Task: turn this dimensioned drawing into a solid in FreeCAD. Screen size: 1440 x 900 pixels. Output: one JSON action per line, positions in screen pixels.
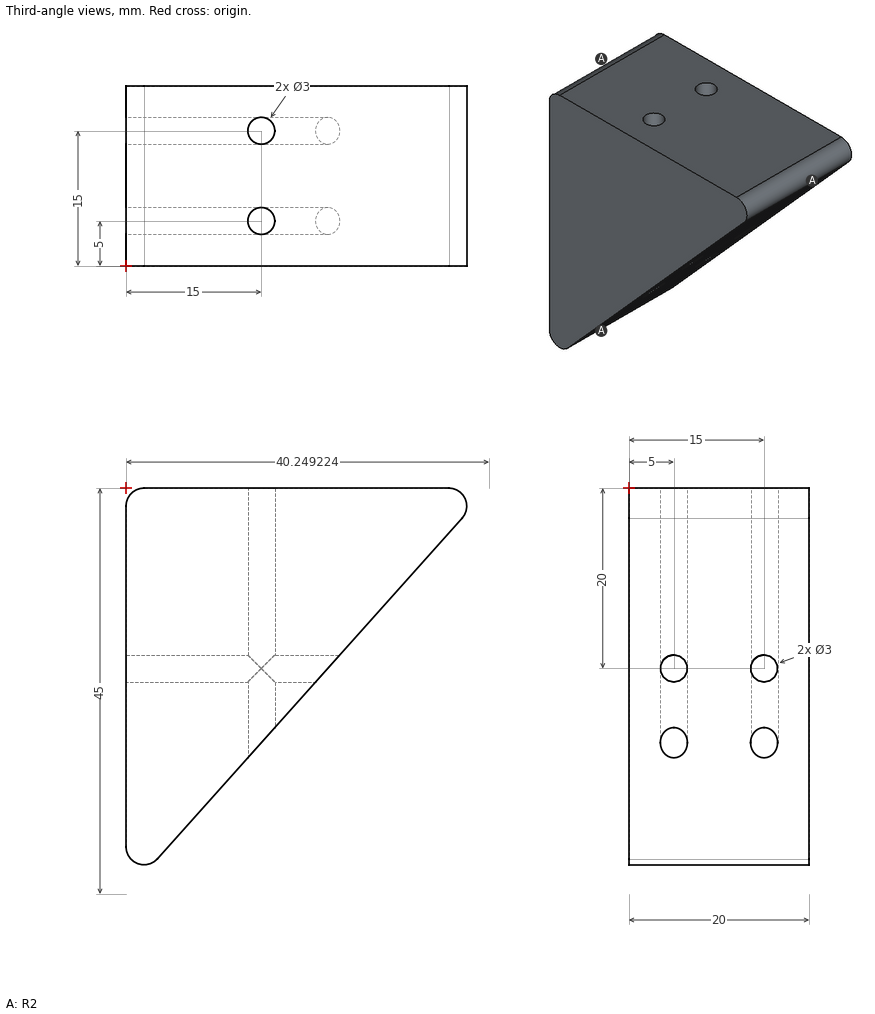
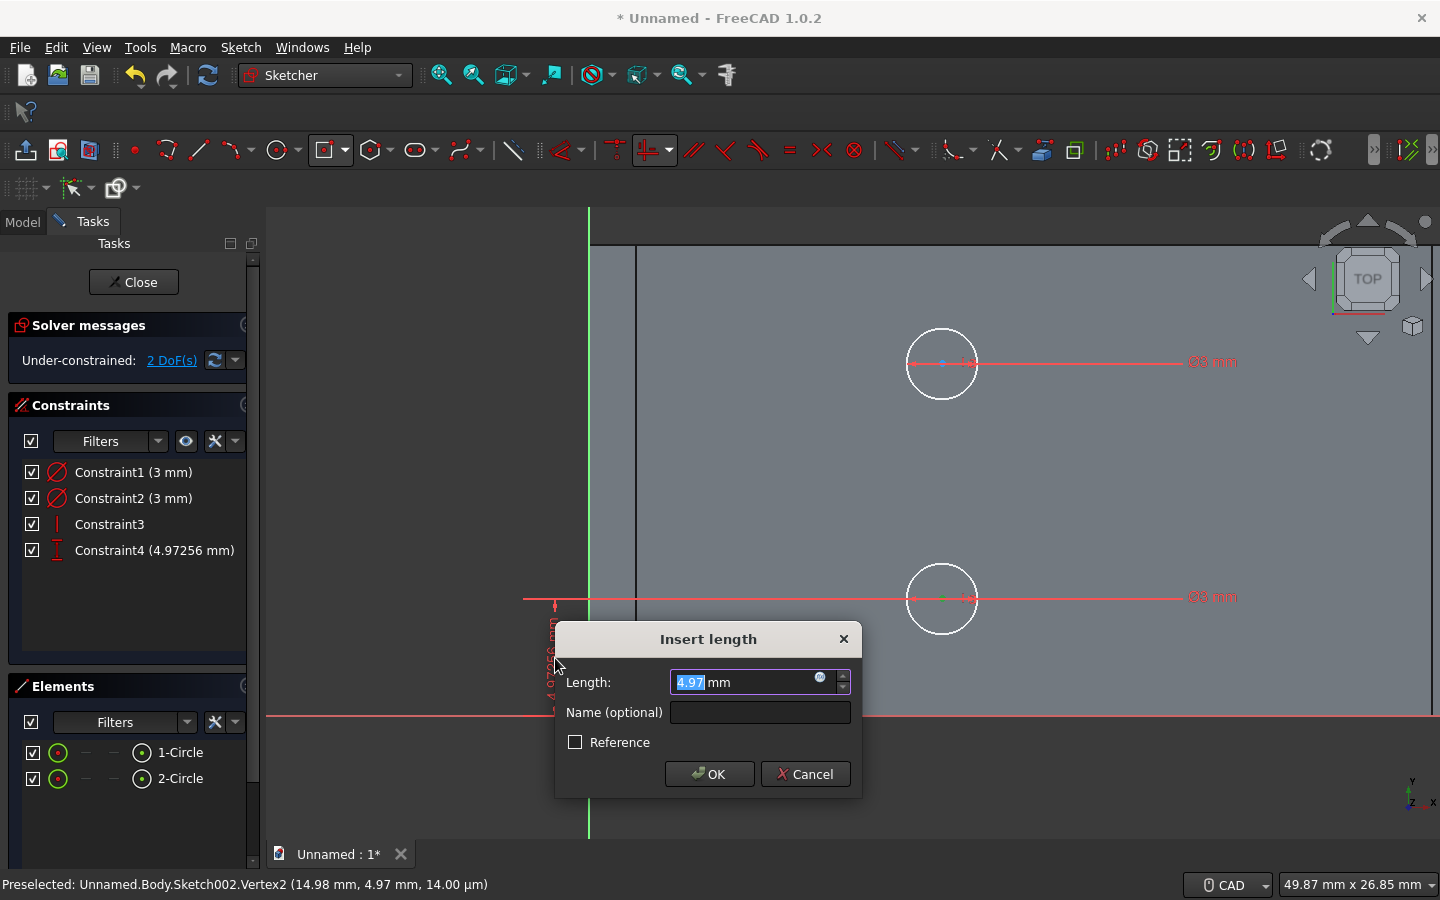
{"action": "type", "text": "5"}
{"action": "key", "text": "Return"}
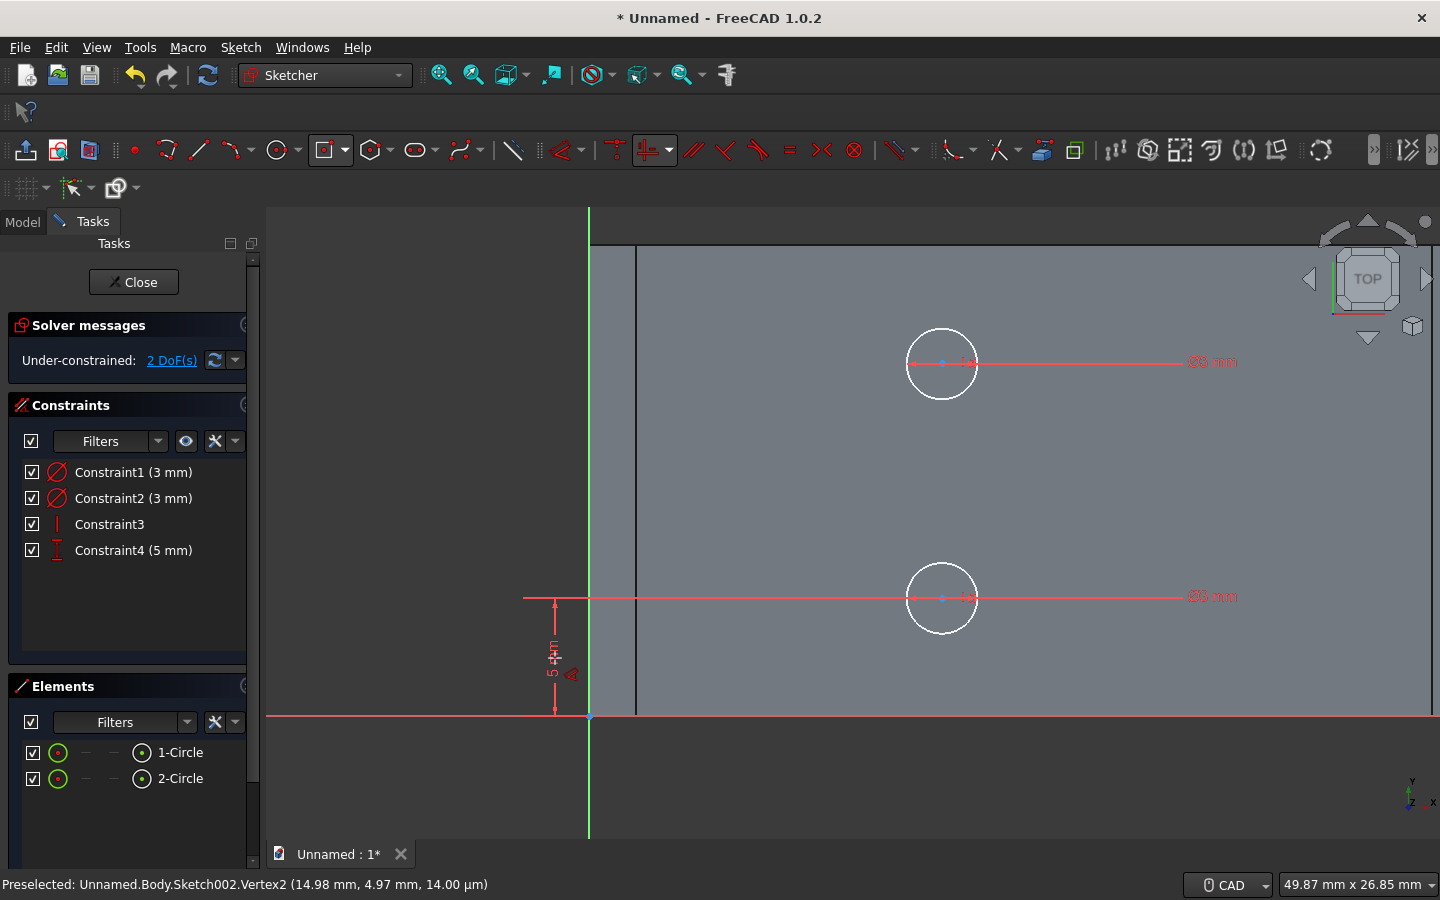
{"action": "left_click", "coordinate": [942, 364]}
{"action": "left_click", "coordinate": [766, 750]}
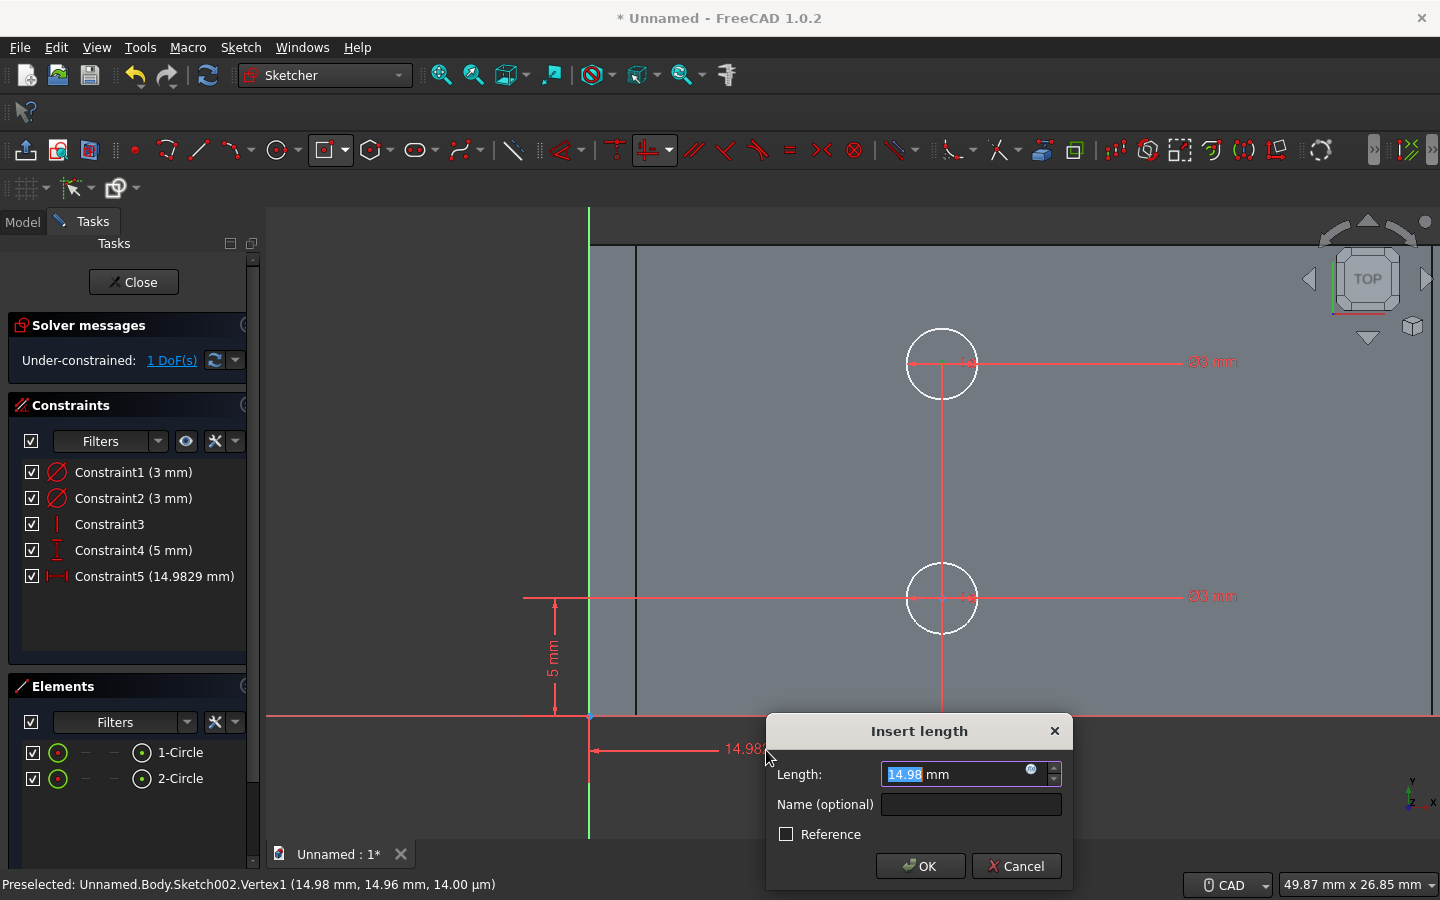
{"action": "type", "text": "15"}
{"action": "key", "text": "Return"}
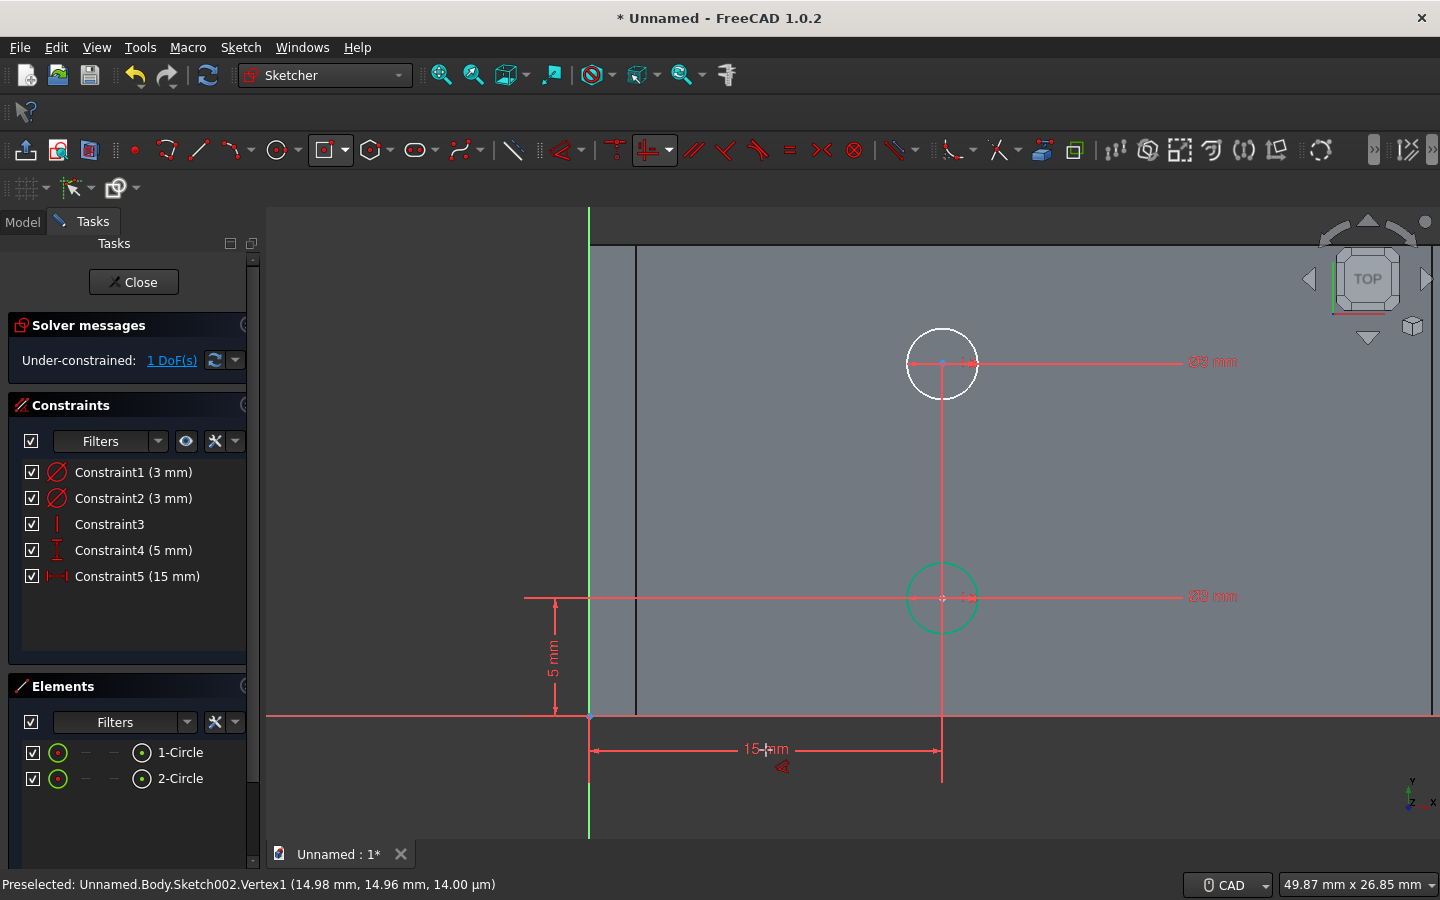
{"action": "left_click", "coordinate": [942, 364]}
{"action": "left_click", "coordinate": [555, 540]}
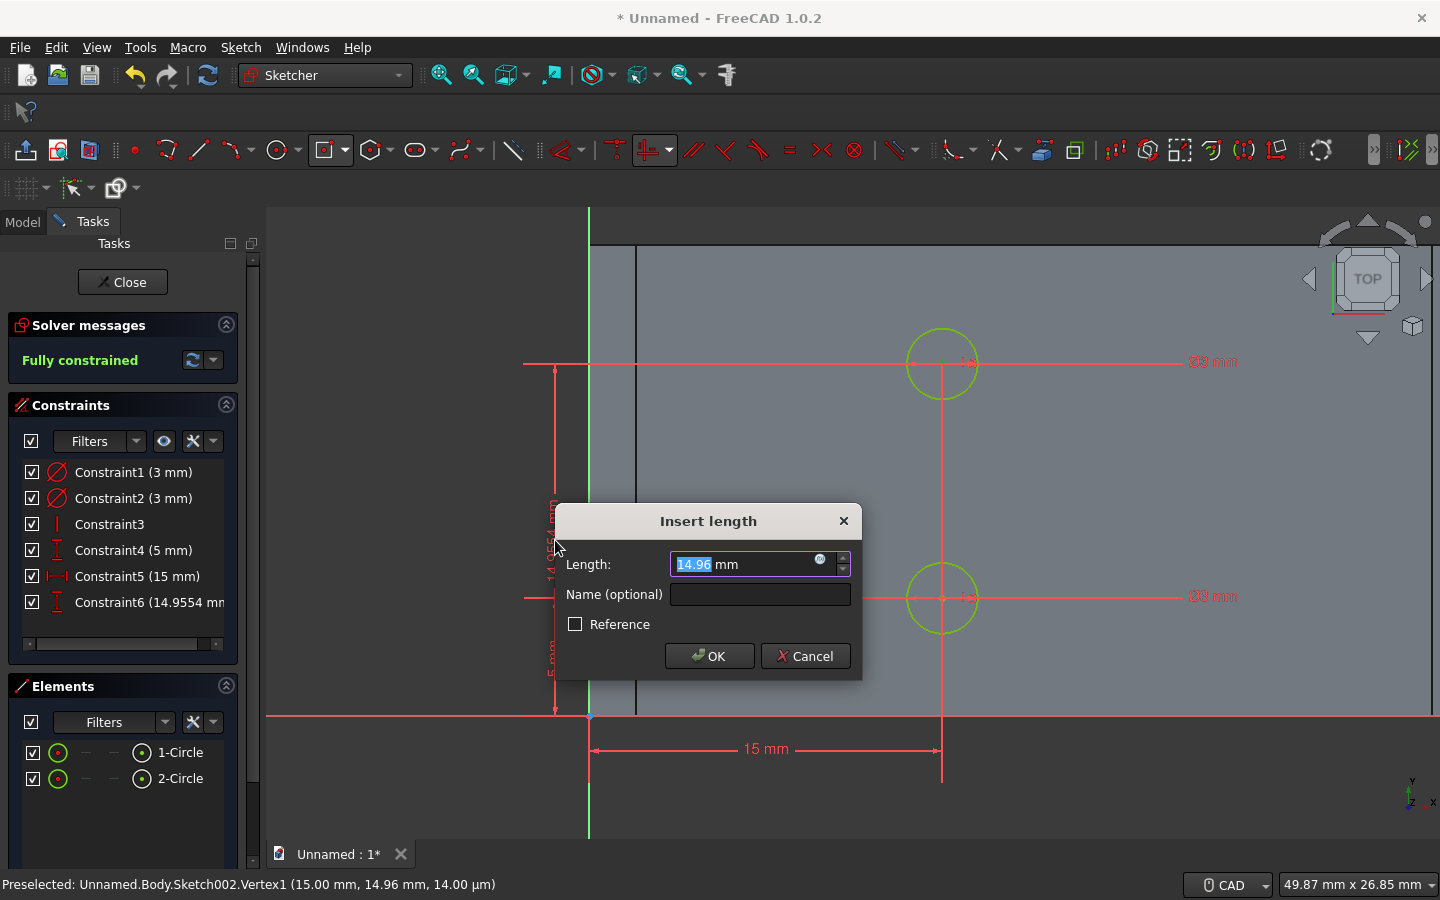
{"action": "type", "text": "15"}
{"action": "key", "text": "Return"}
{"action": "key", "text": "Escape"}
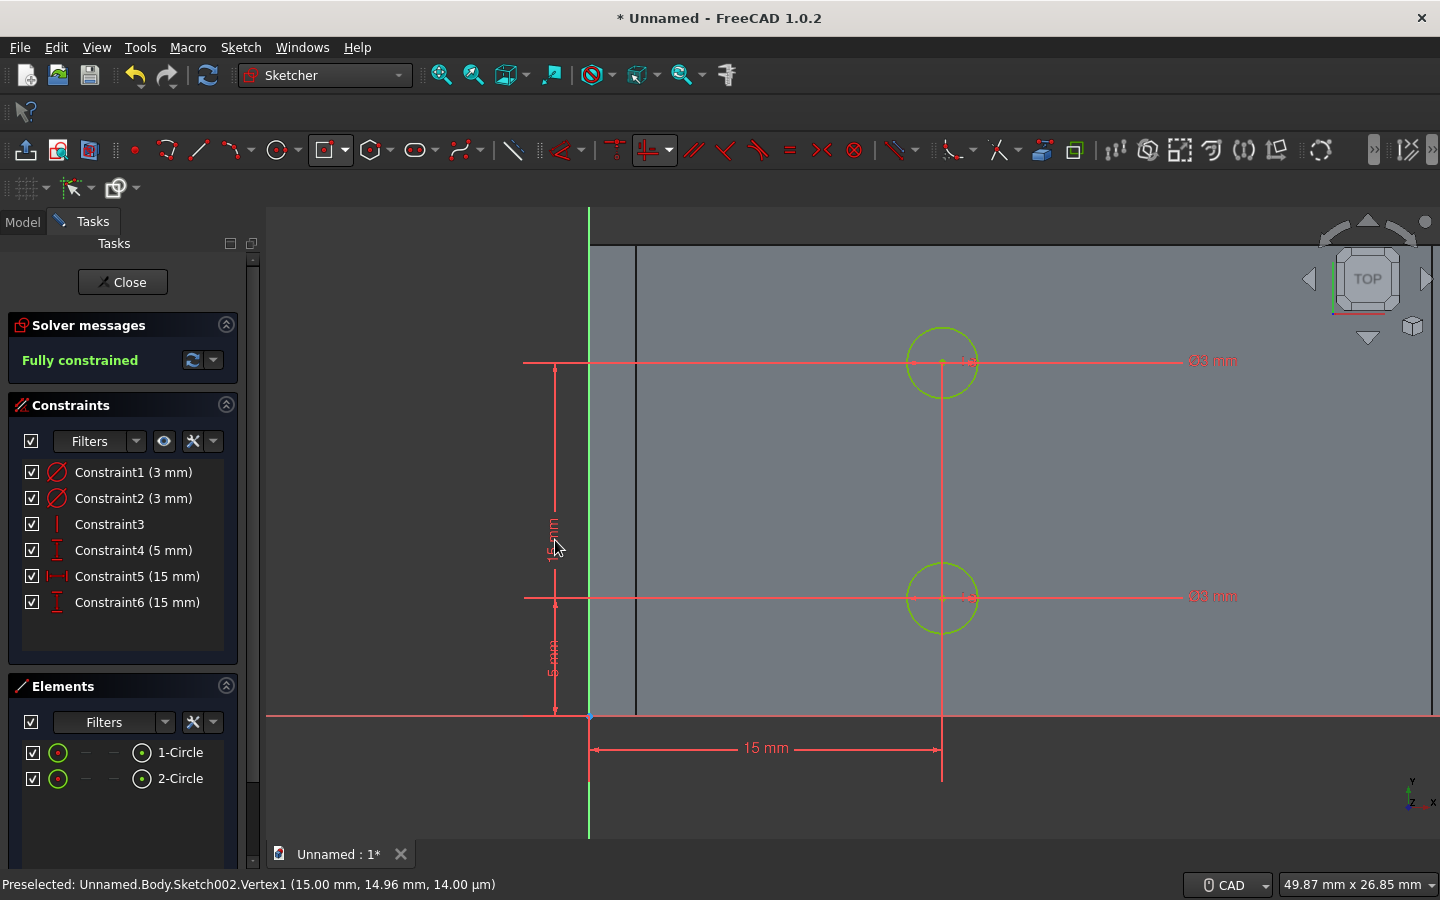
{"action": "left_click", "coordinate": [123, 282]}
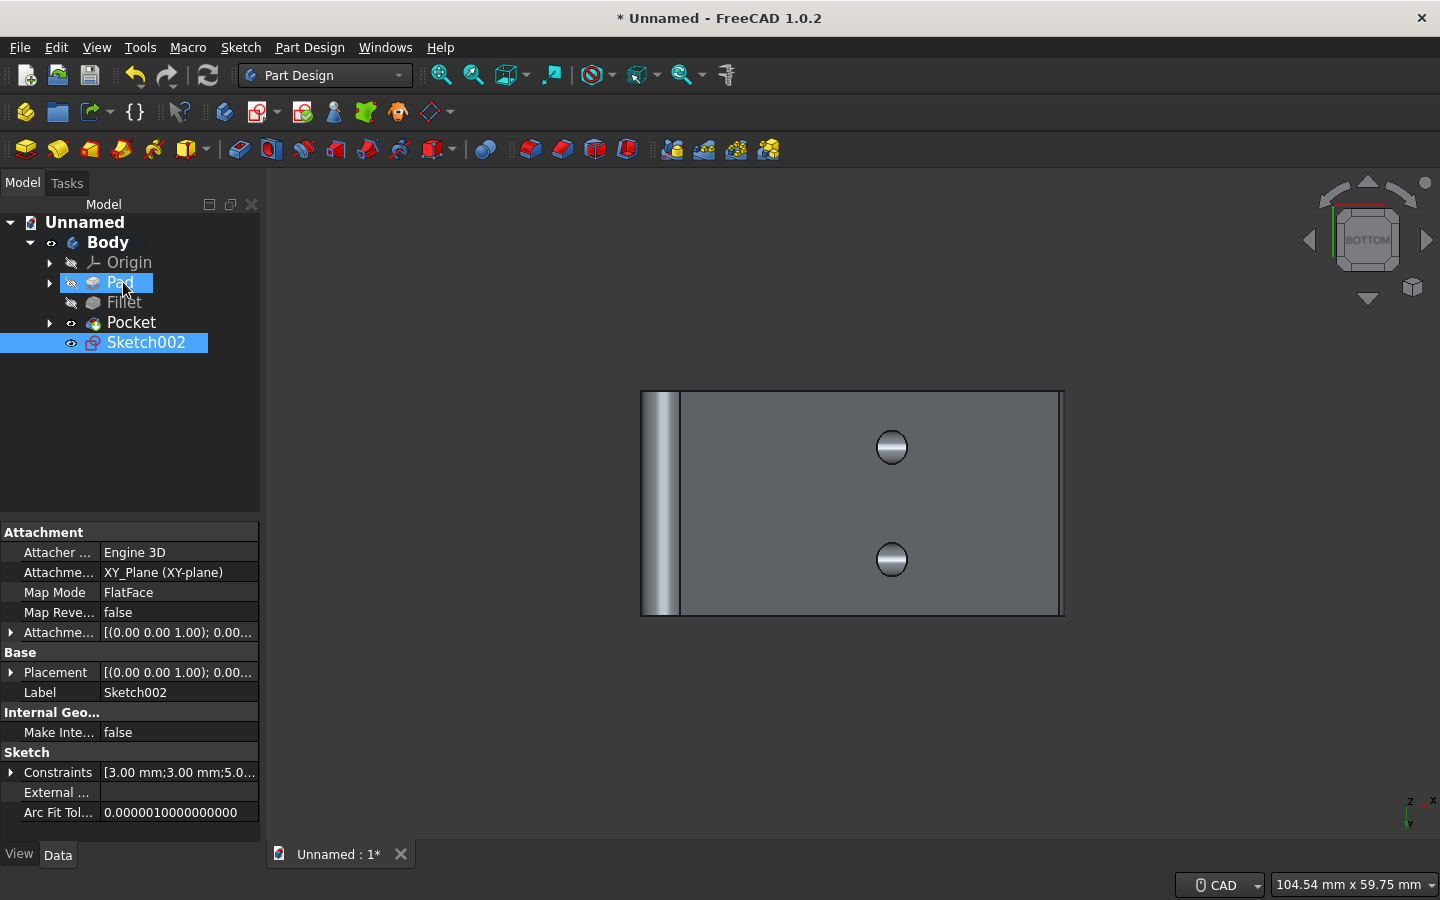
{"action": "left_click", "coordinate": [240, 150]}